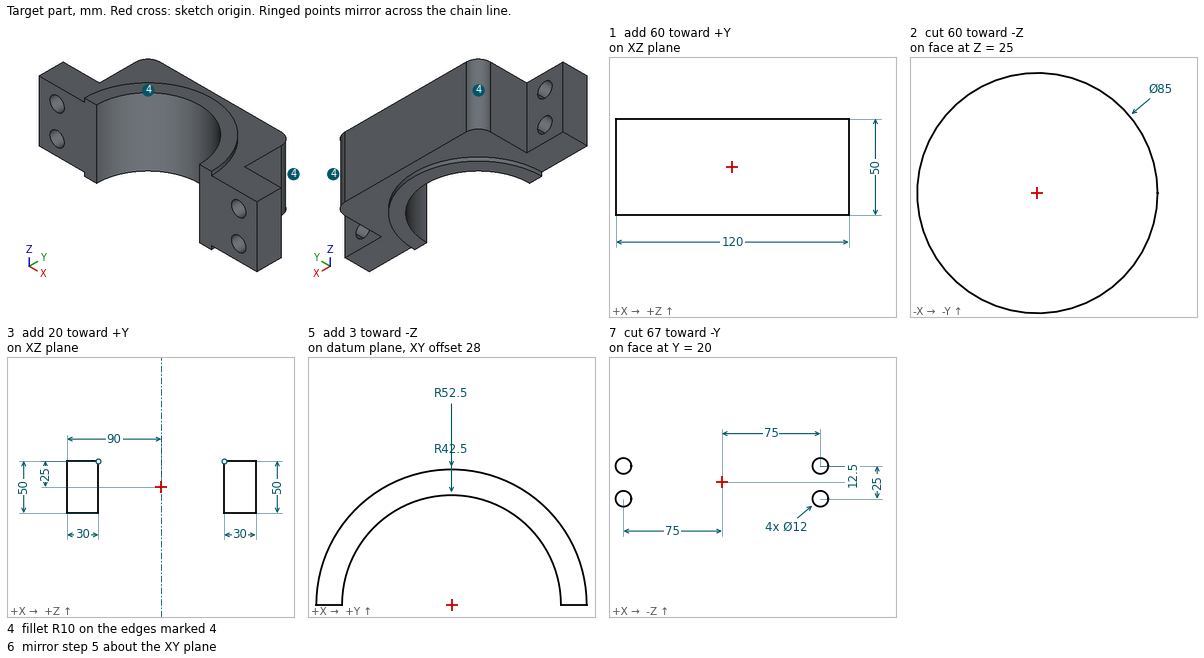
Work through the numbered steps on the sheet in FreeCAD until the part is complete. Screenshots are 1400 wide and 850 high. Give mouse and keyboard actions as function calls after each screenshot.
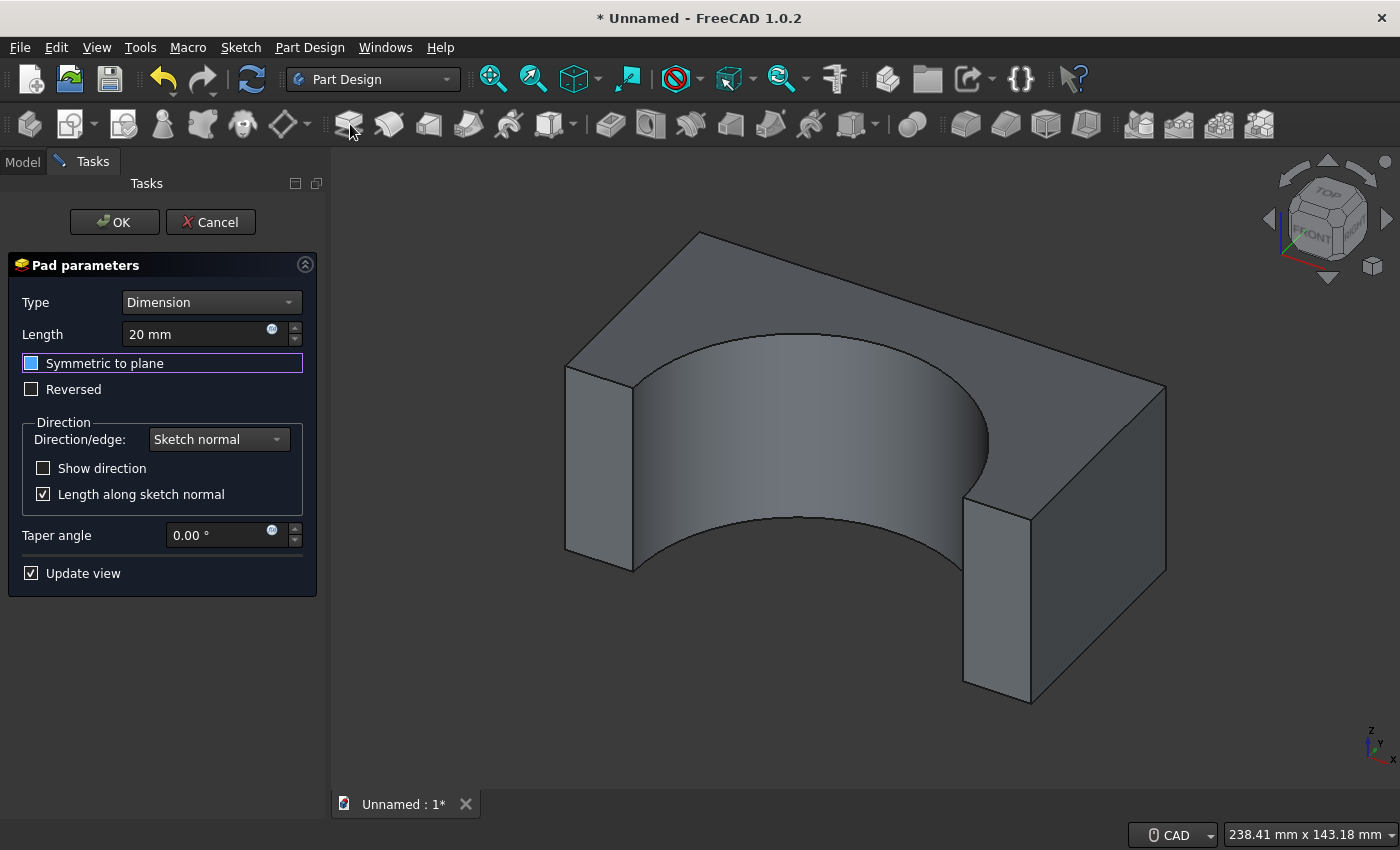
click(30, 389)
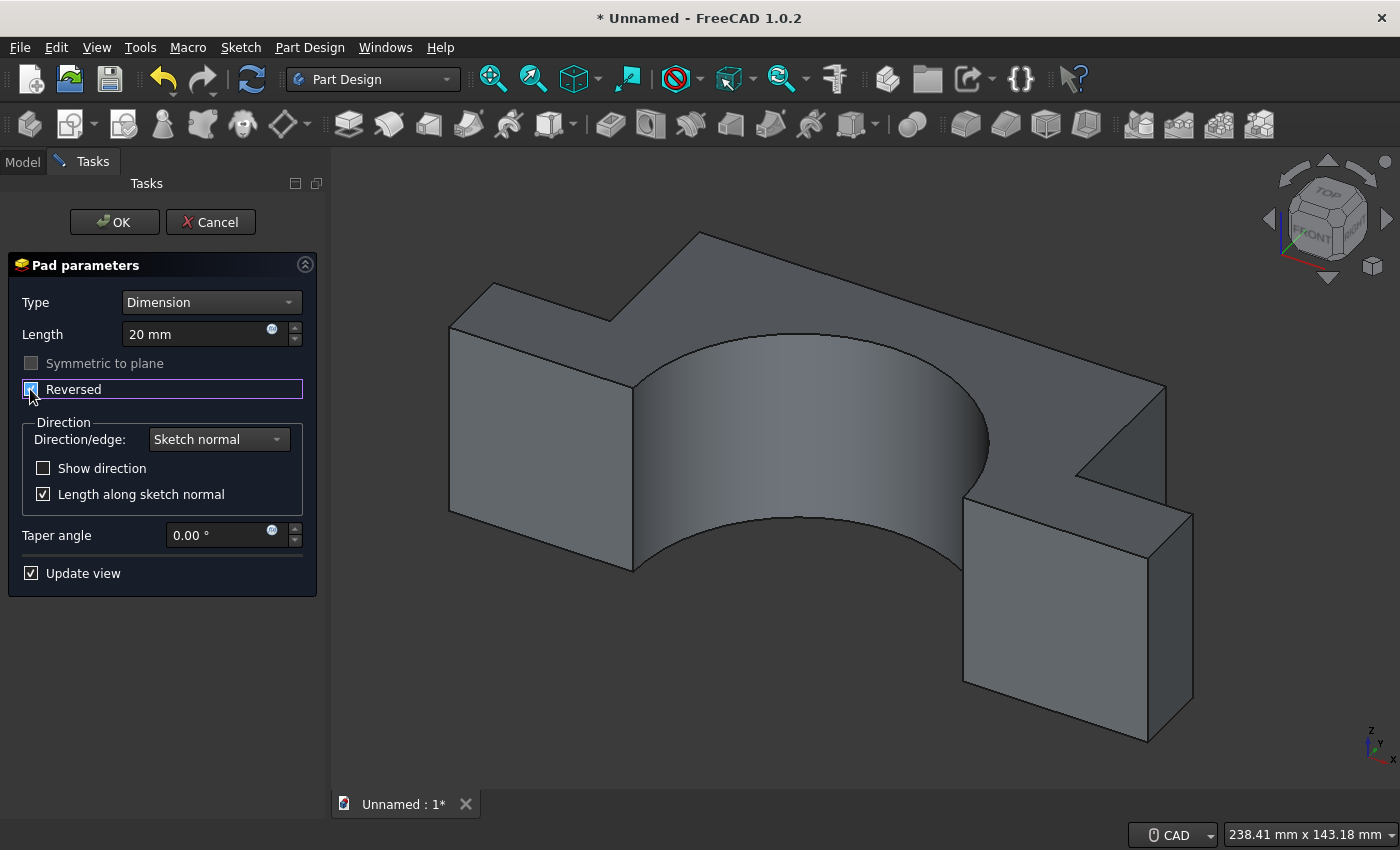
click(115, 222)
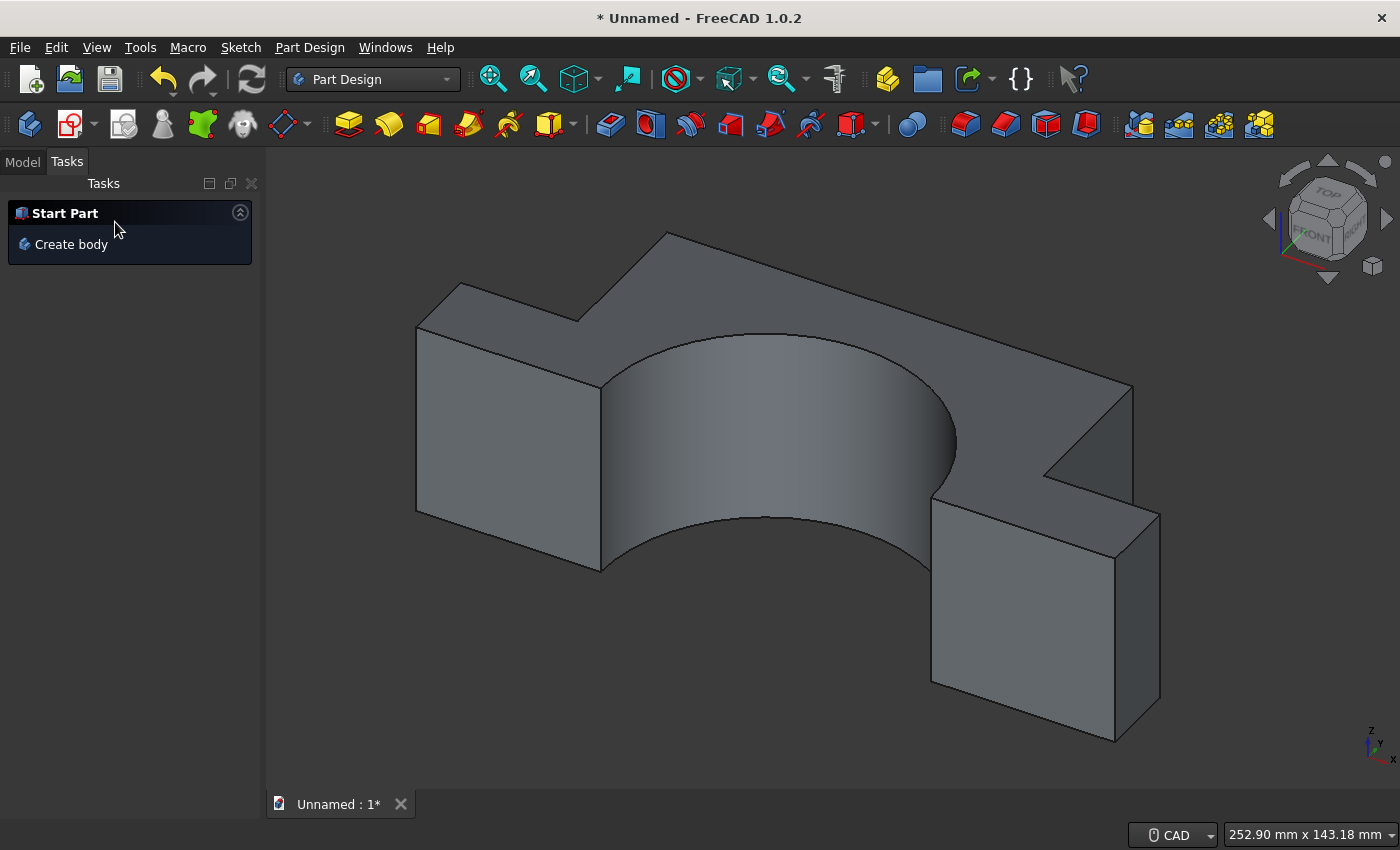
key(0)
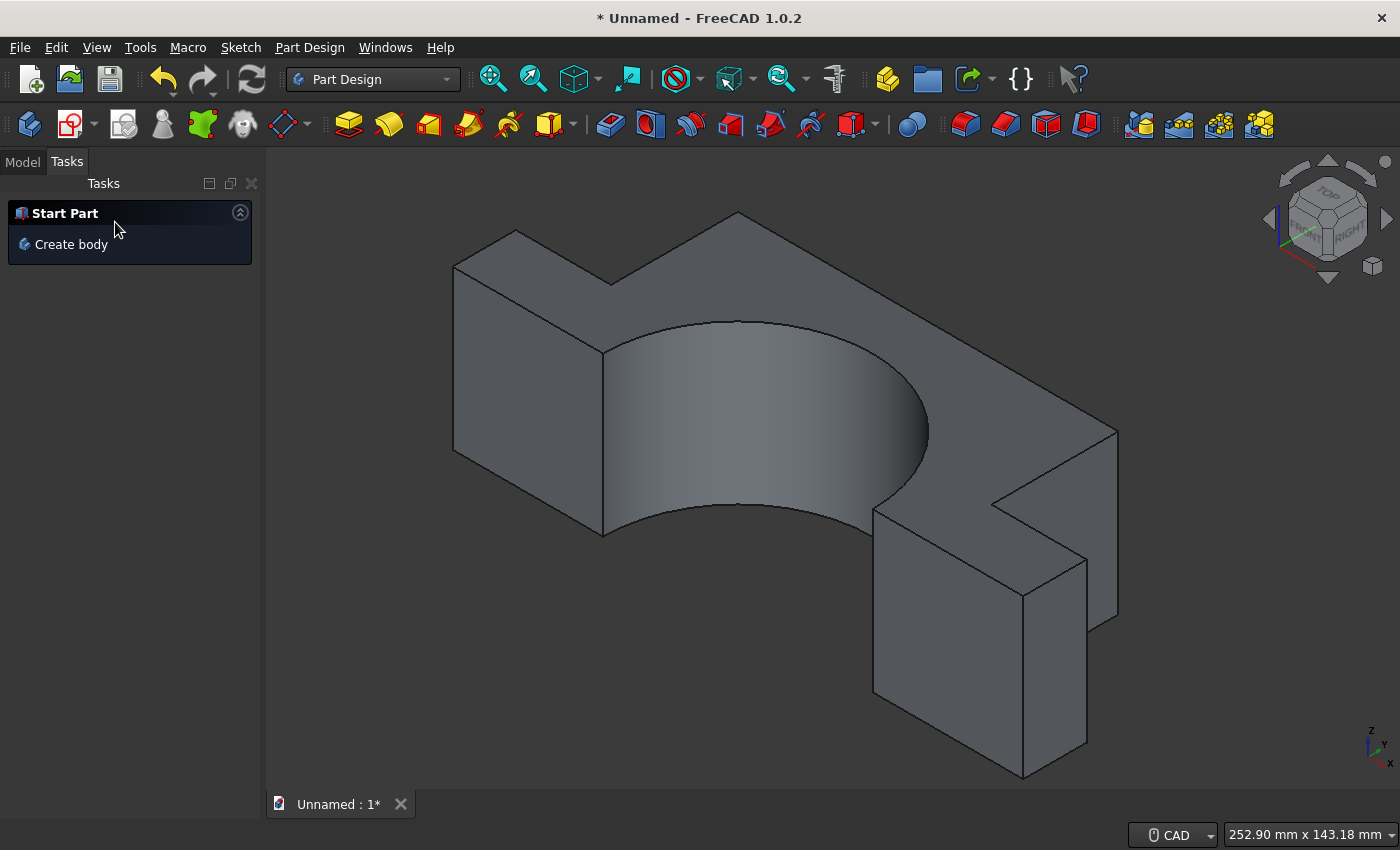
key(2)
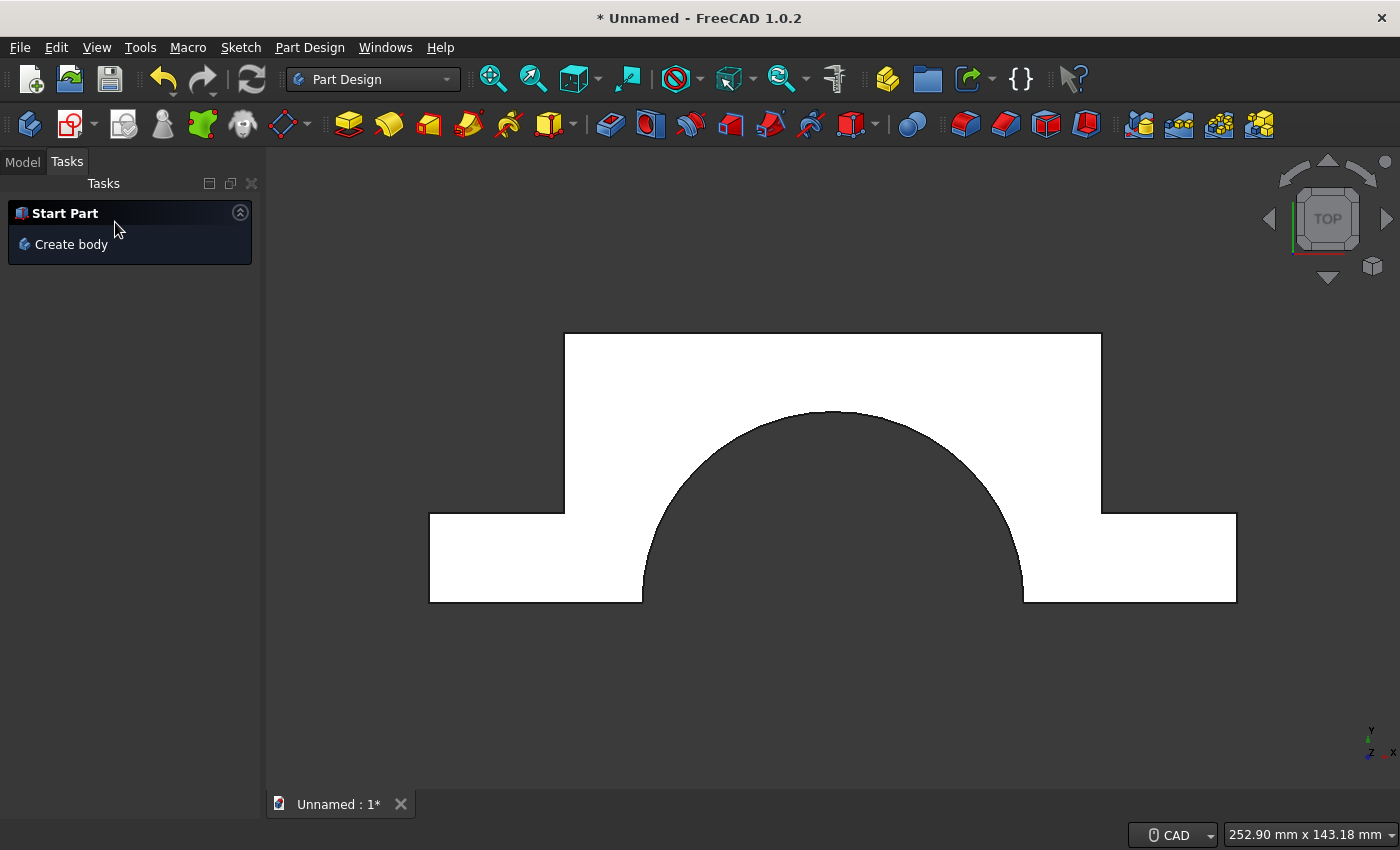
key(1)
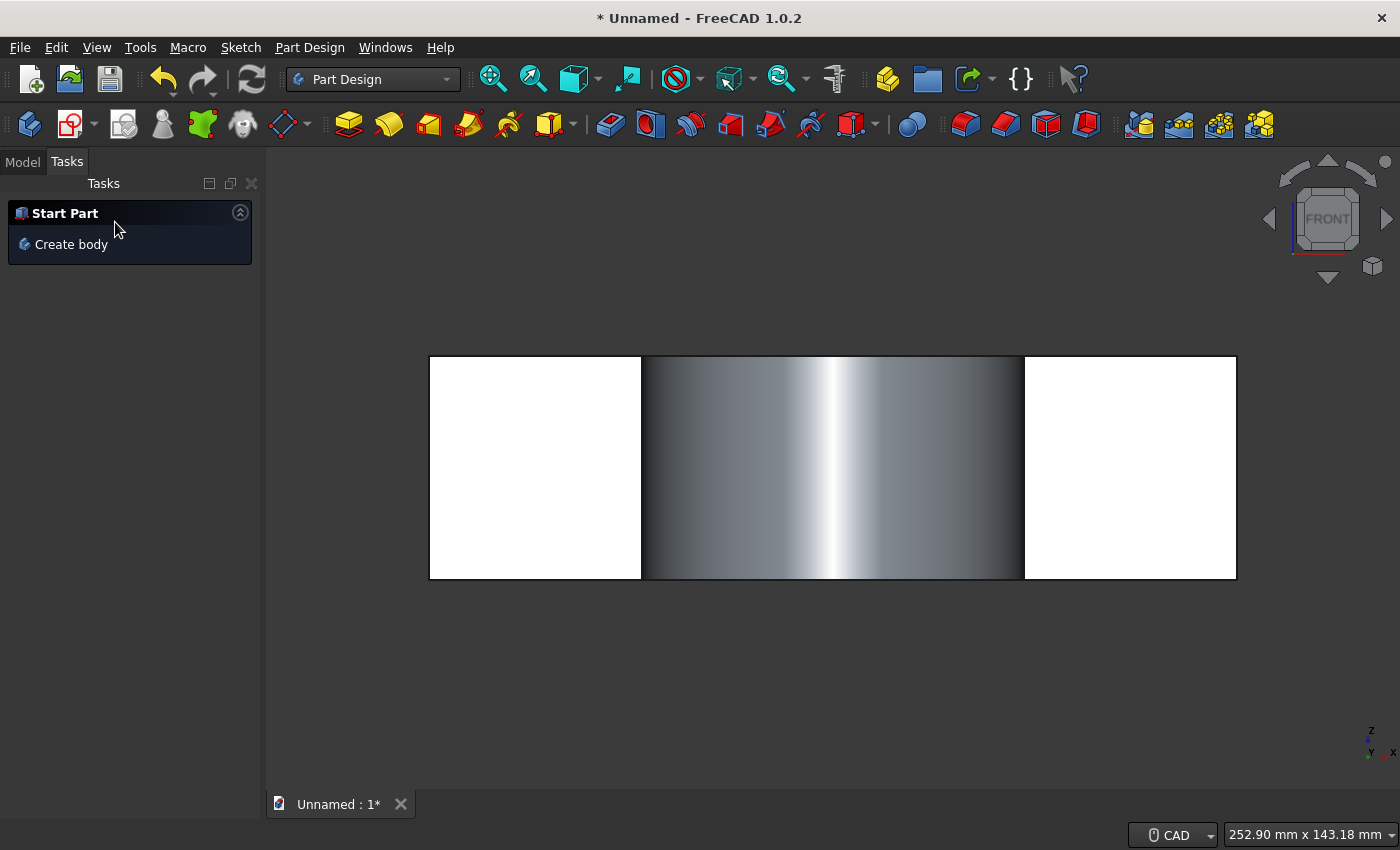
key(3)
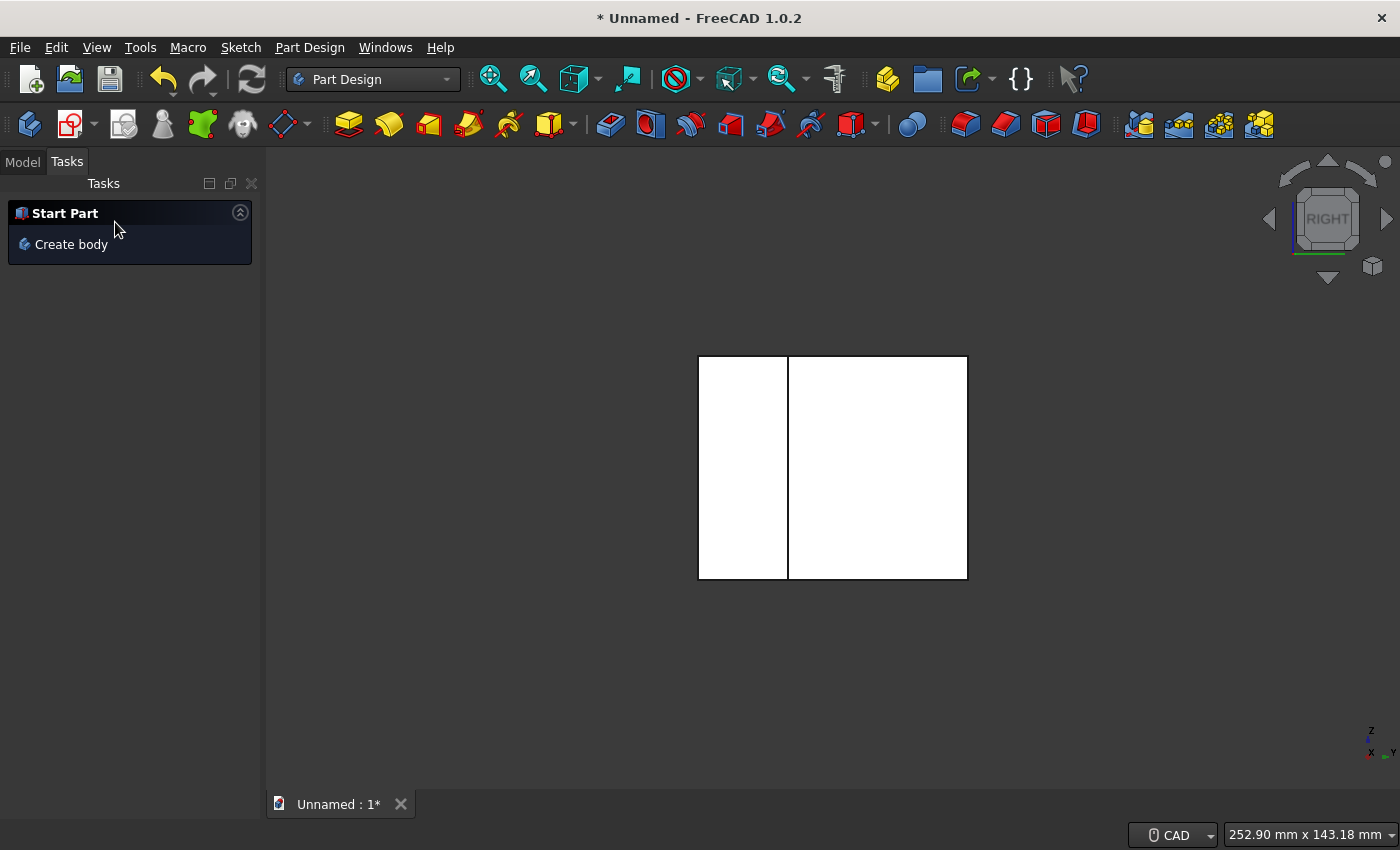
click(494, 80)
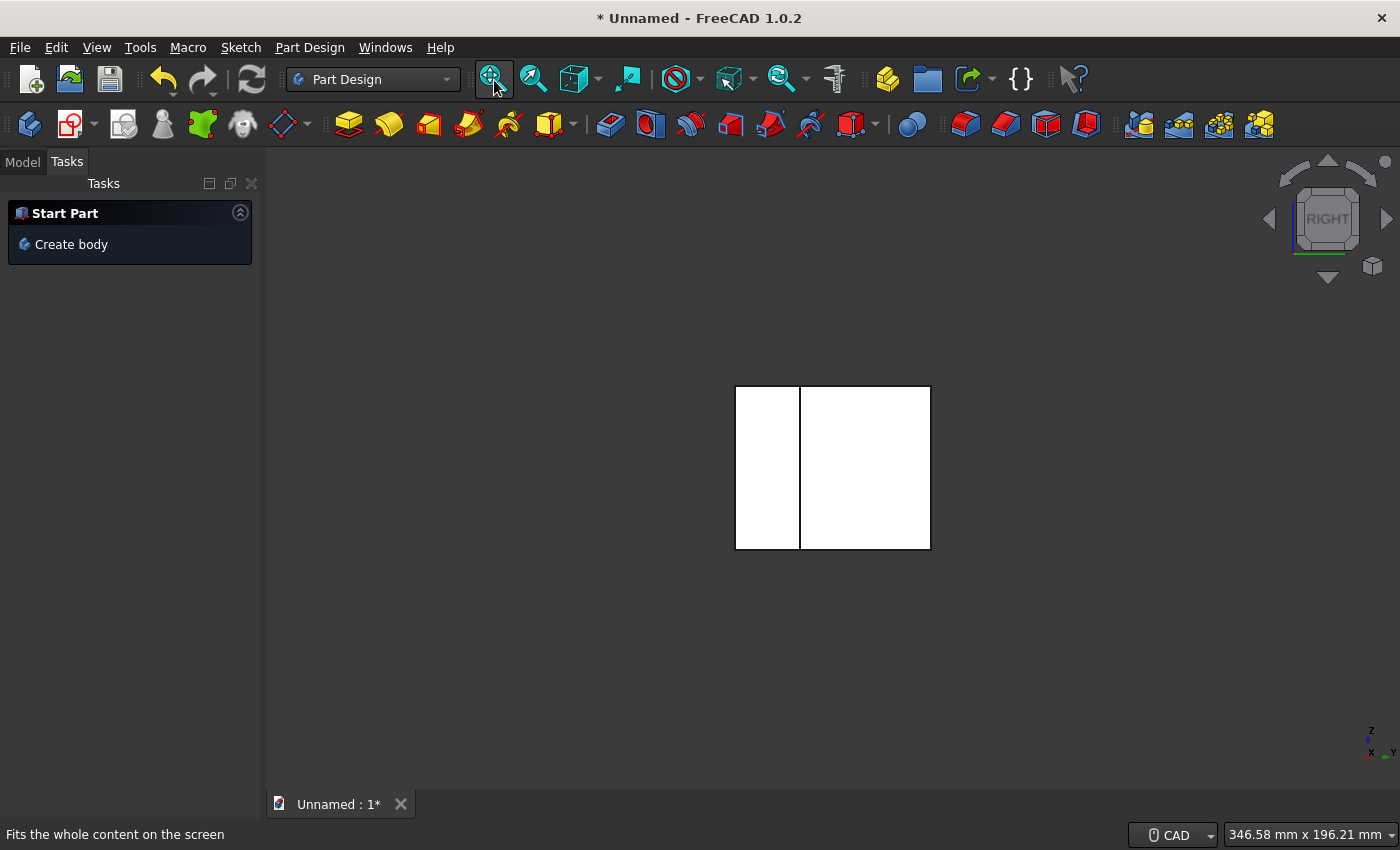
click(931, 467)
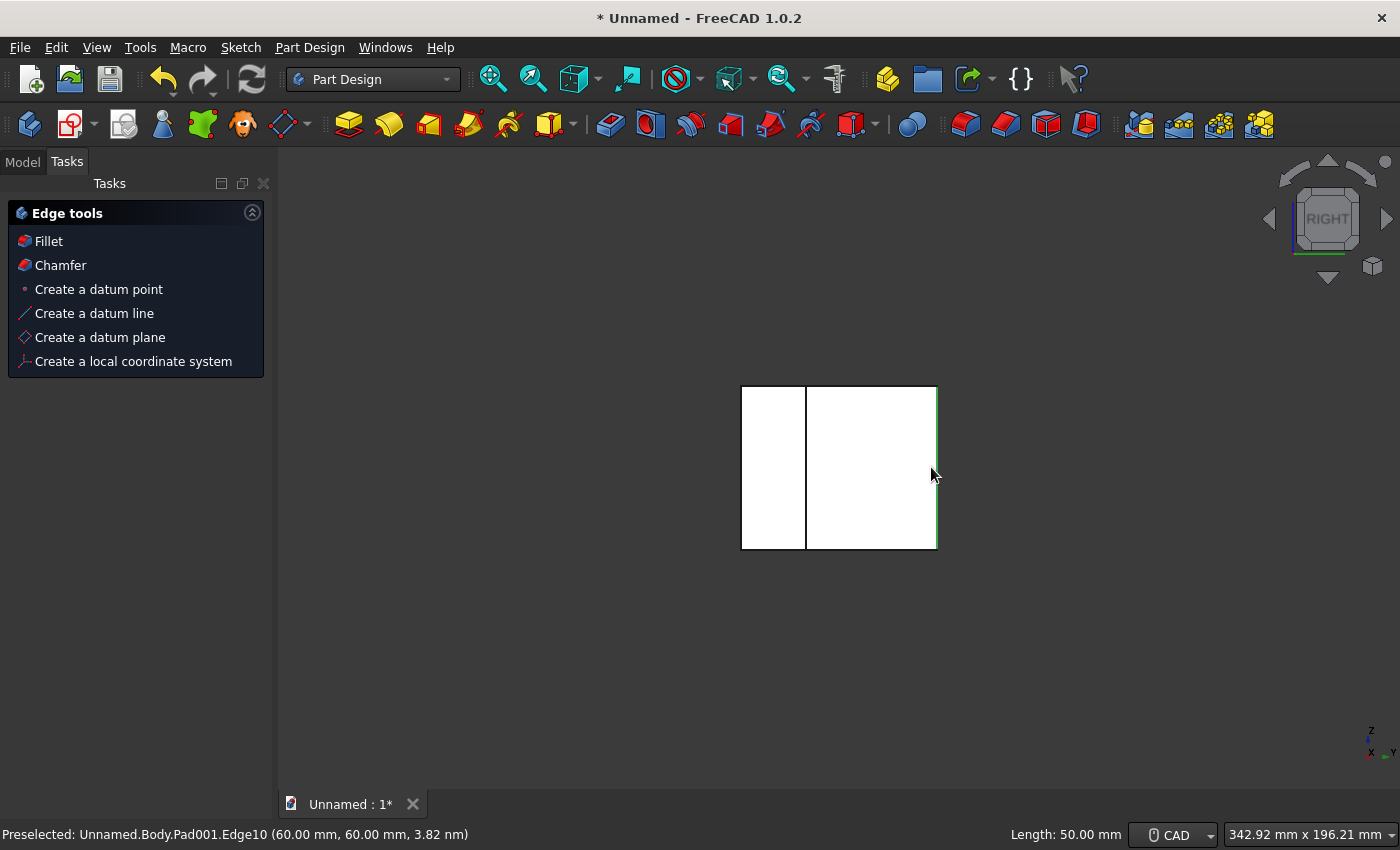
key(5)